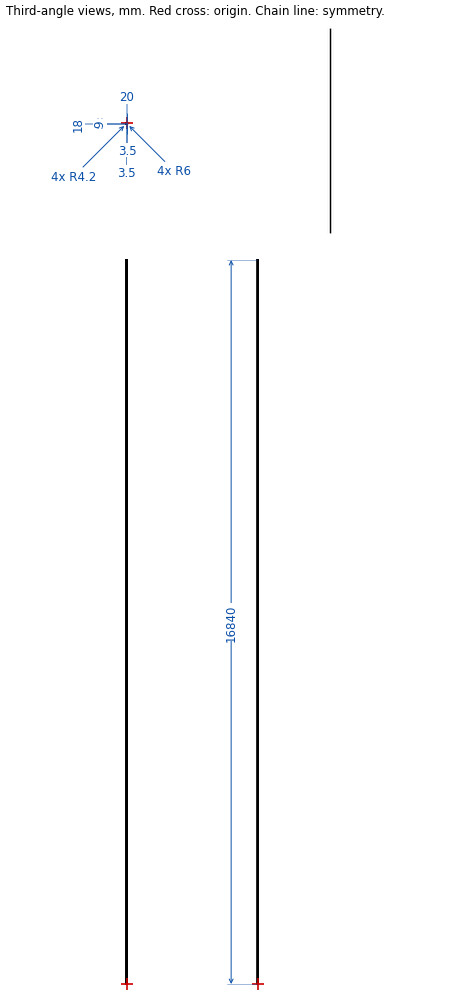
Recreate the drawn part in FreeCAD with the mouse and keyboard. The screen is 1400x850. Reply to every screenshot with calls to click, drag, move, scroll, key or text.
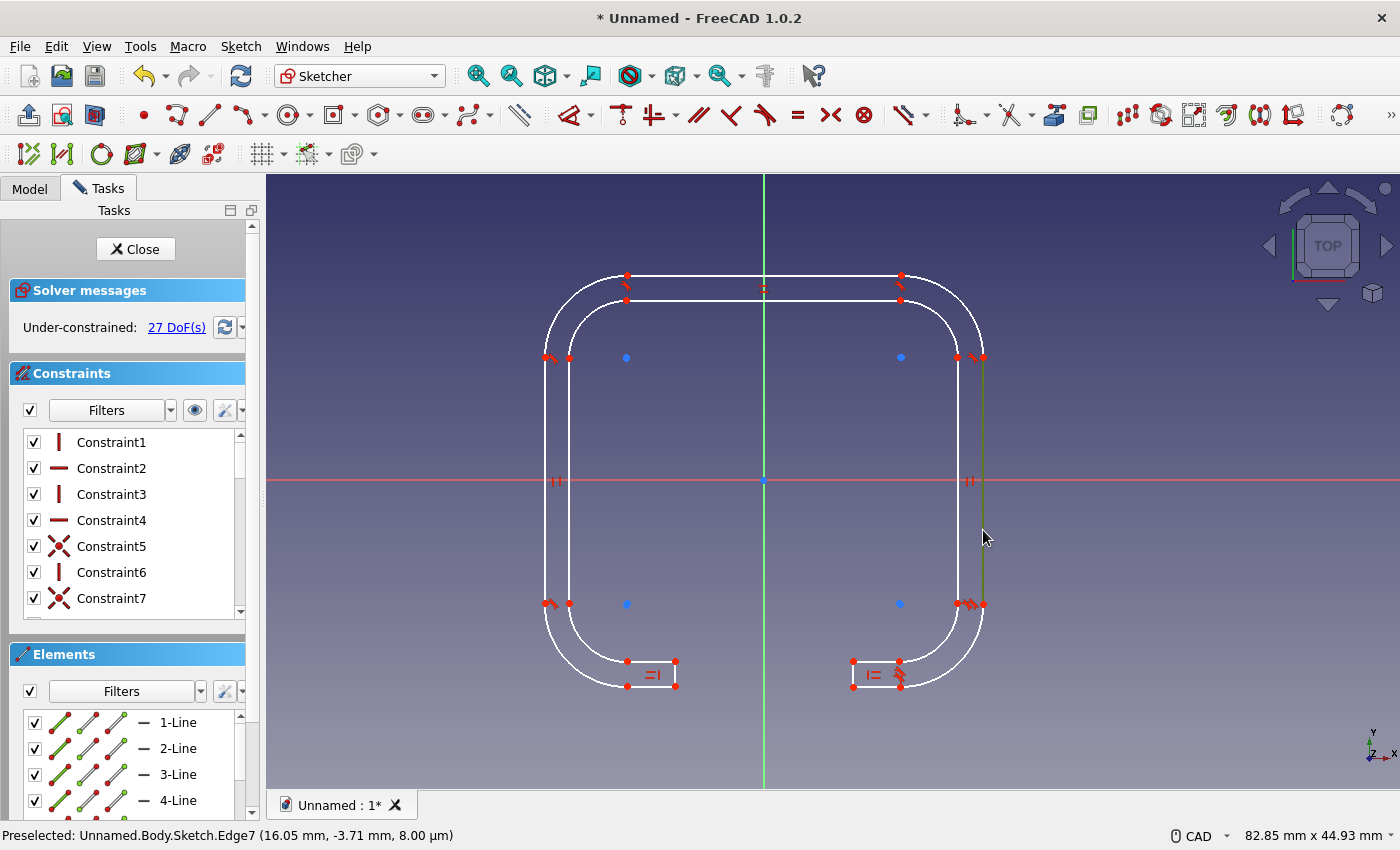
click(974, 321)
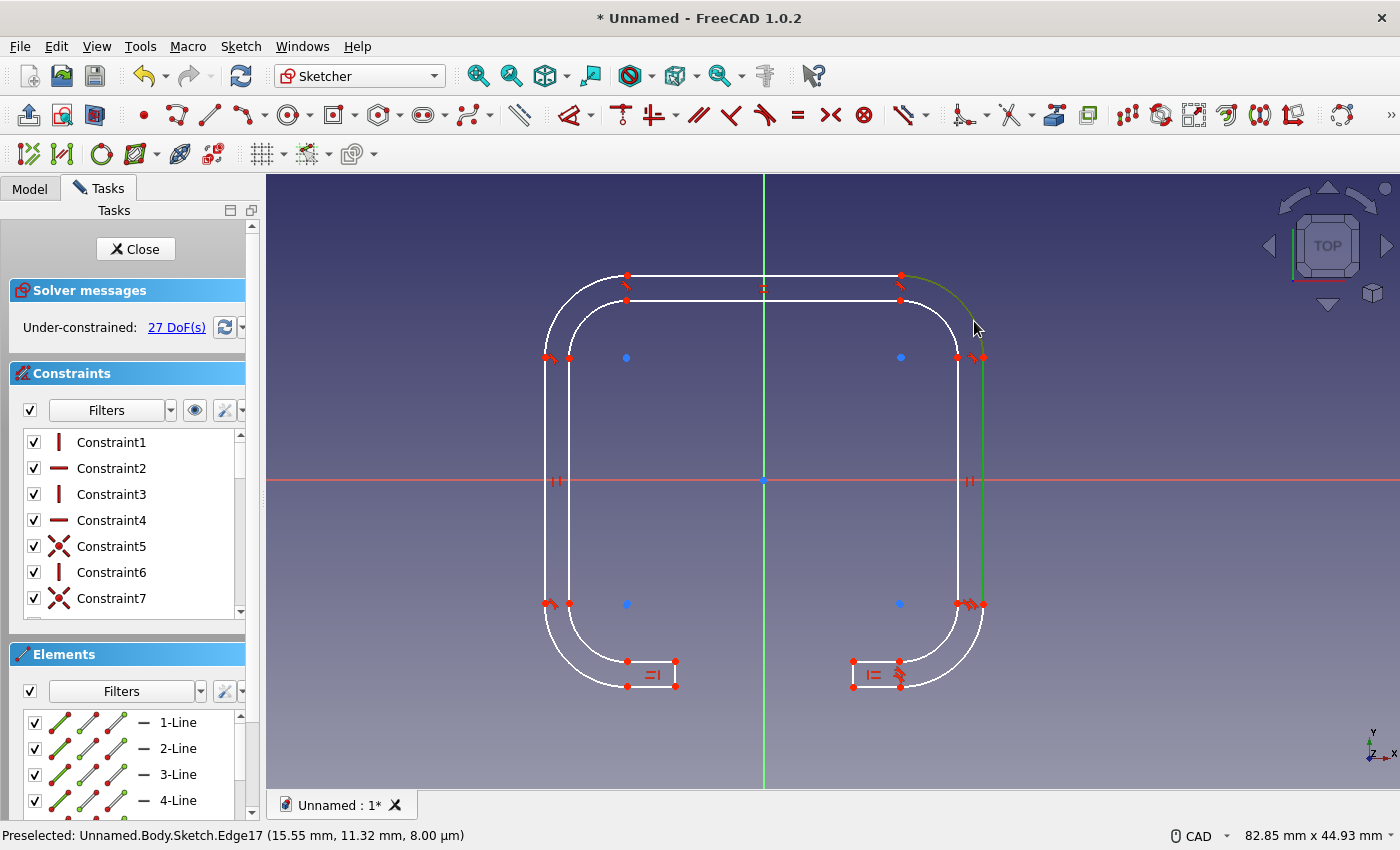
click(765, 116)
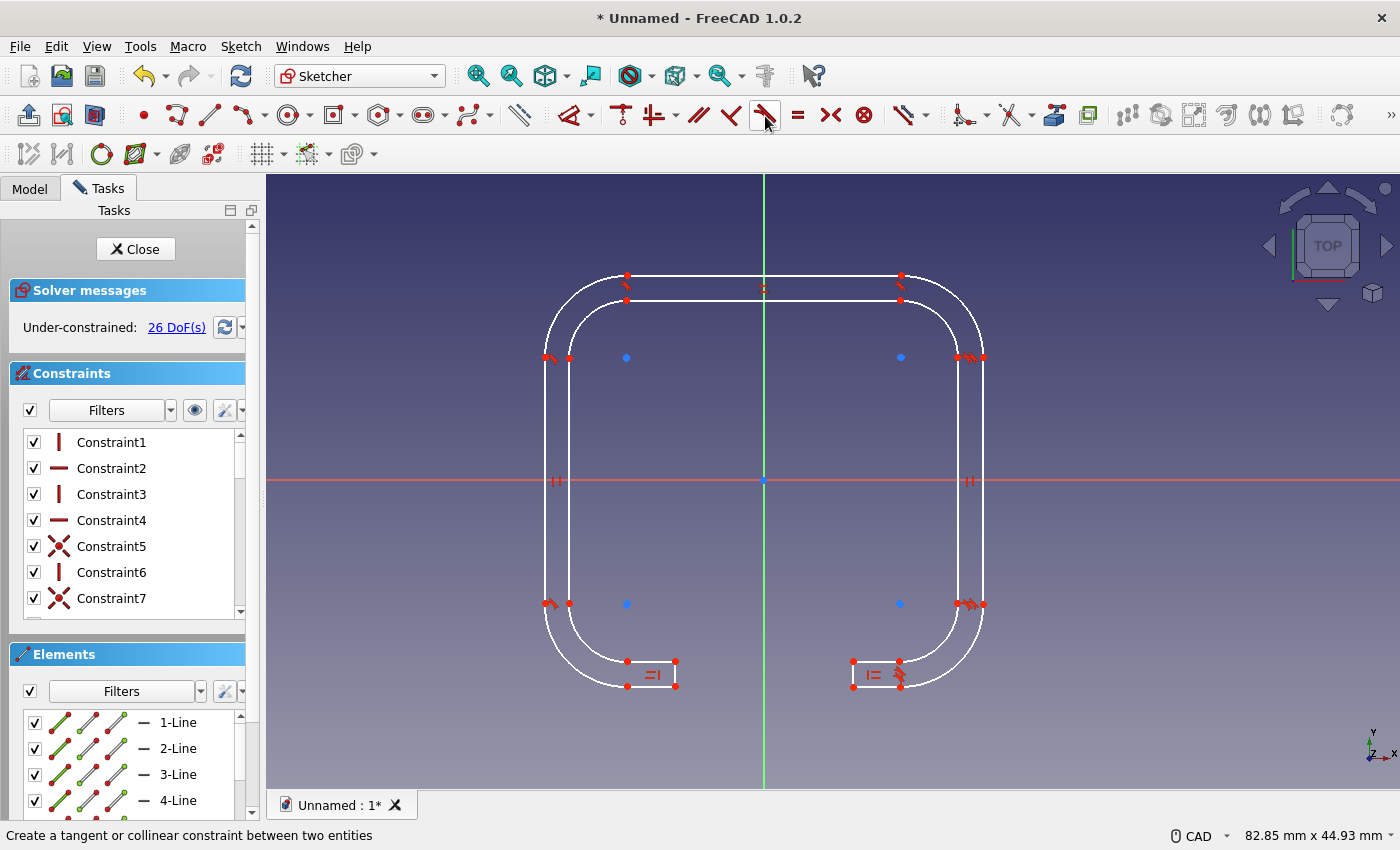
click(819, 276)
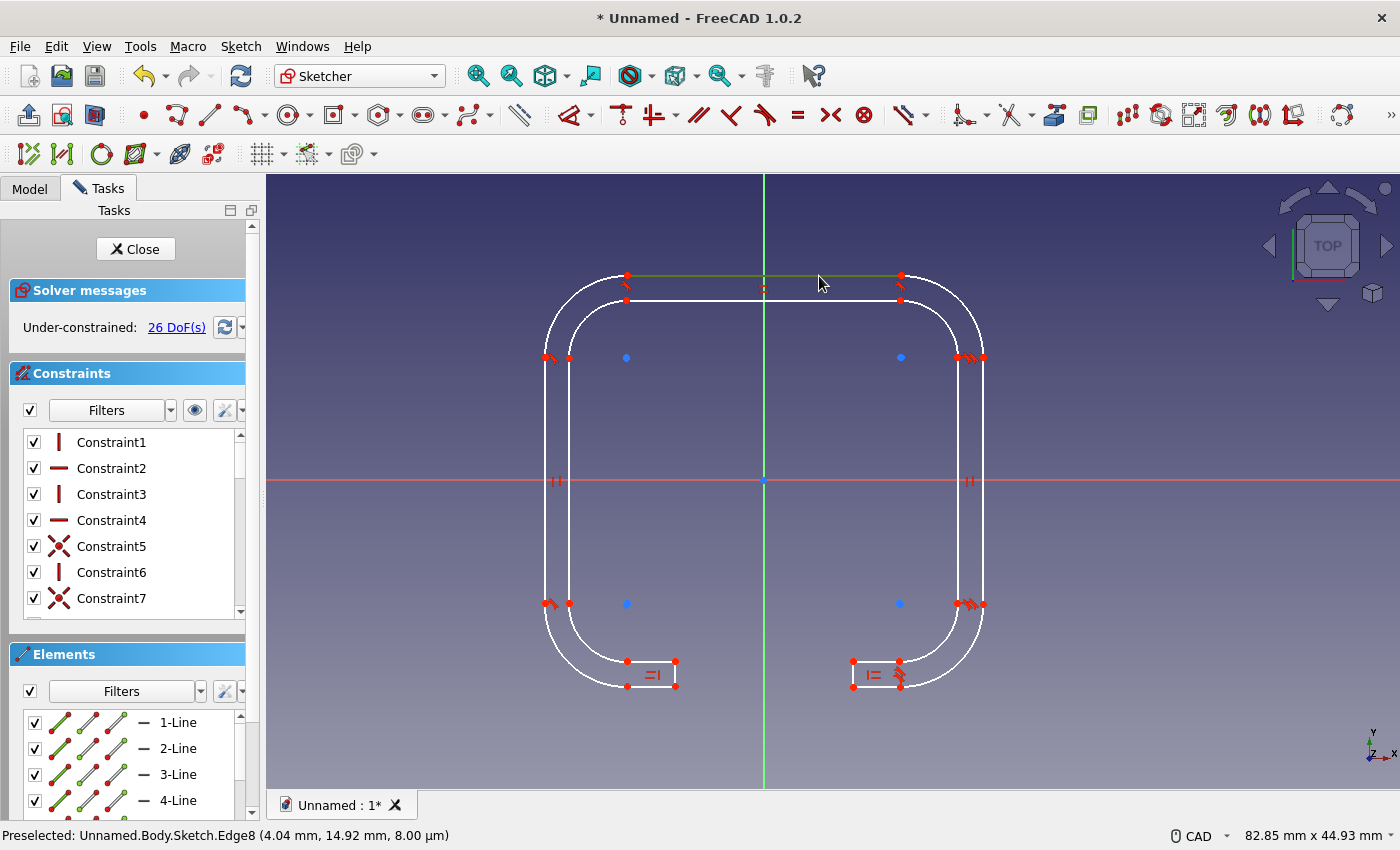
click(974, 321)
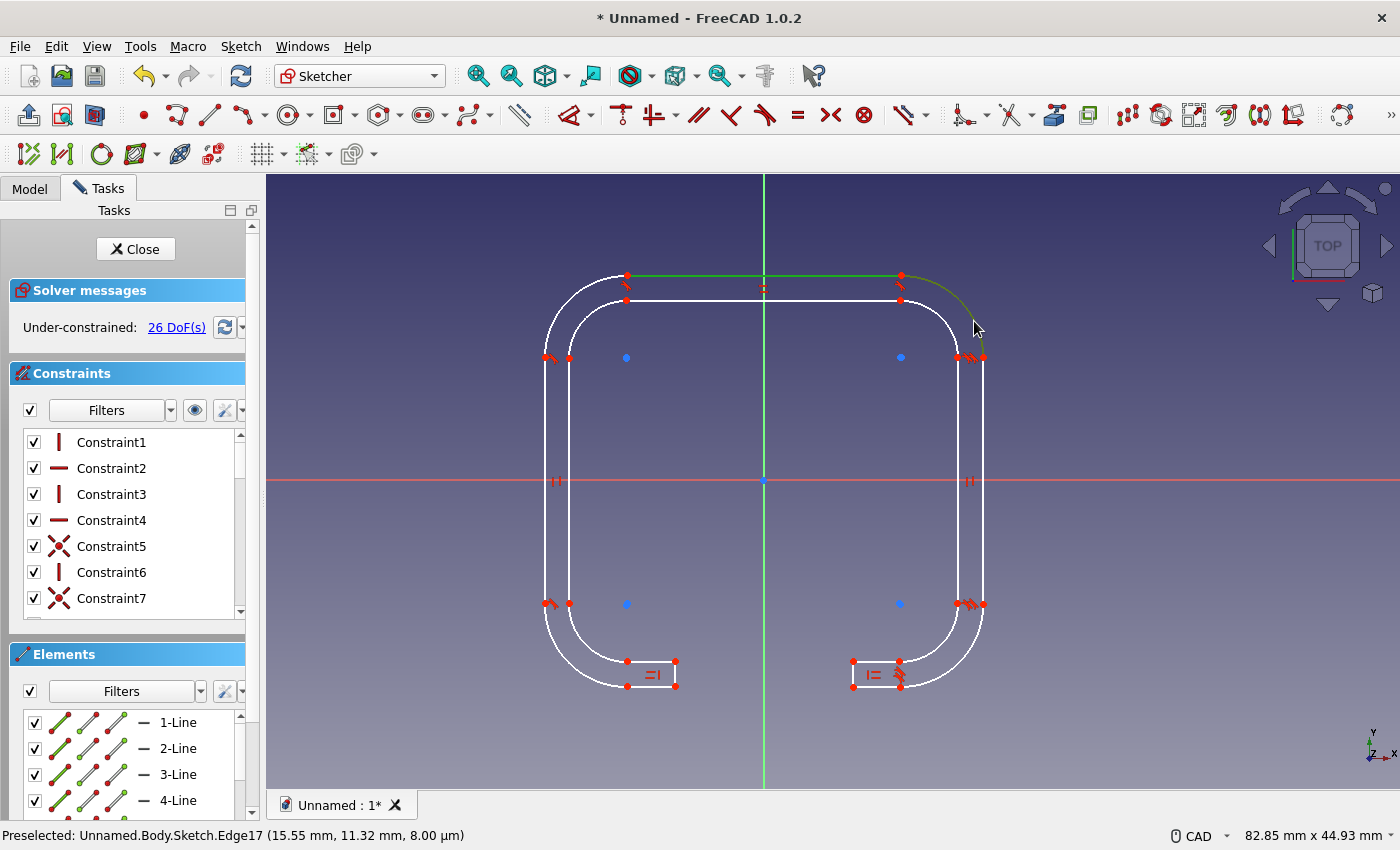
click(765, 116)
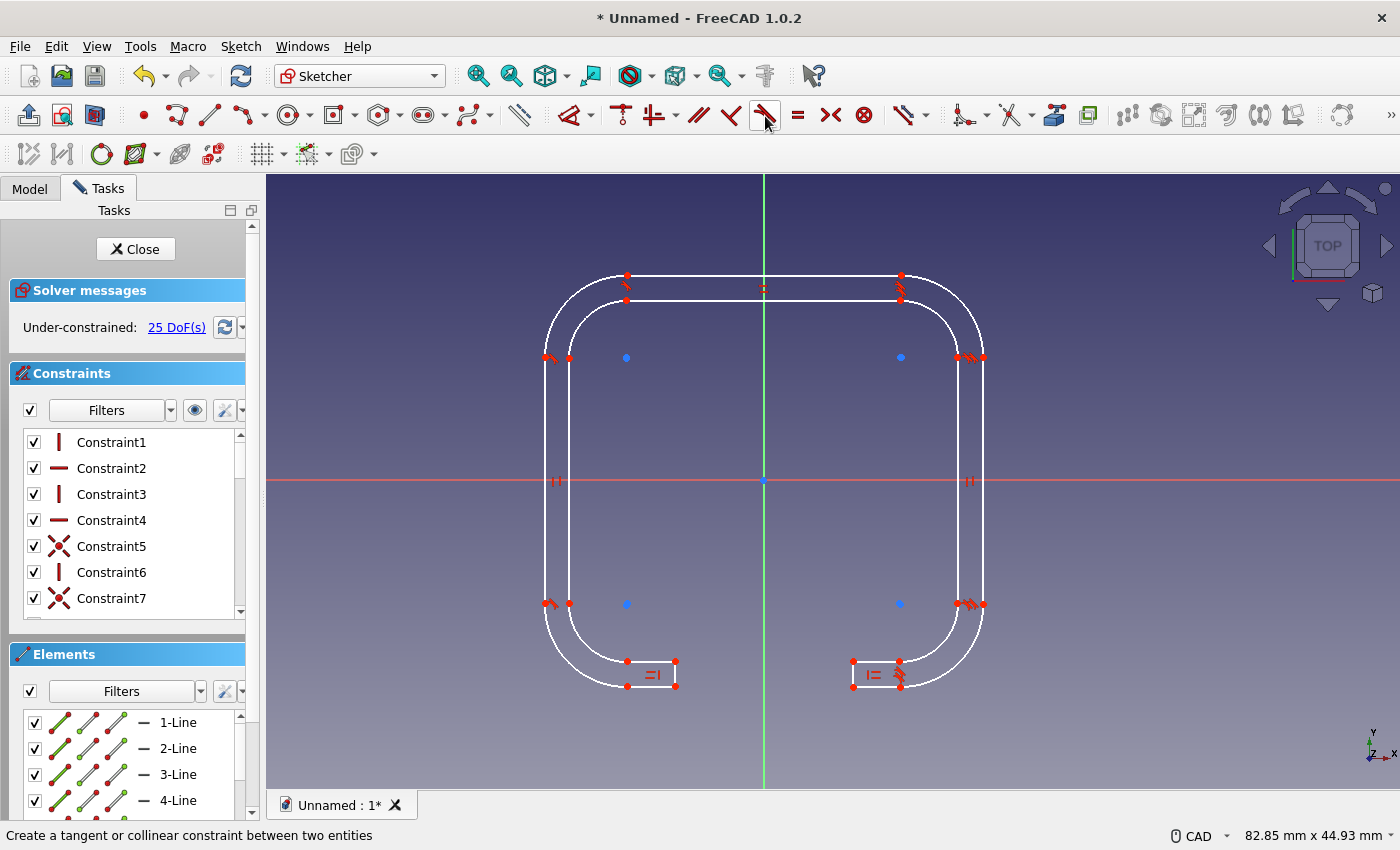
click(819, 276)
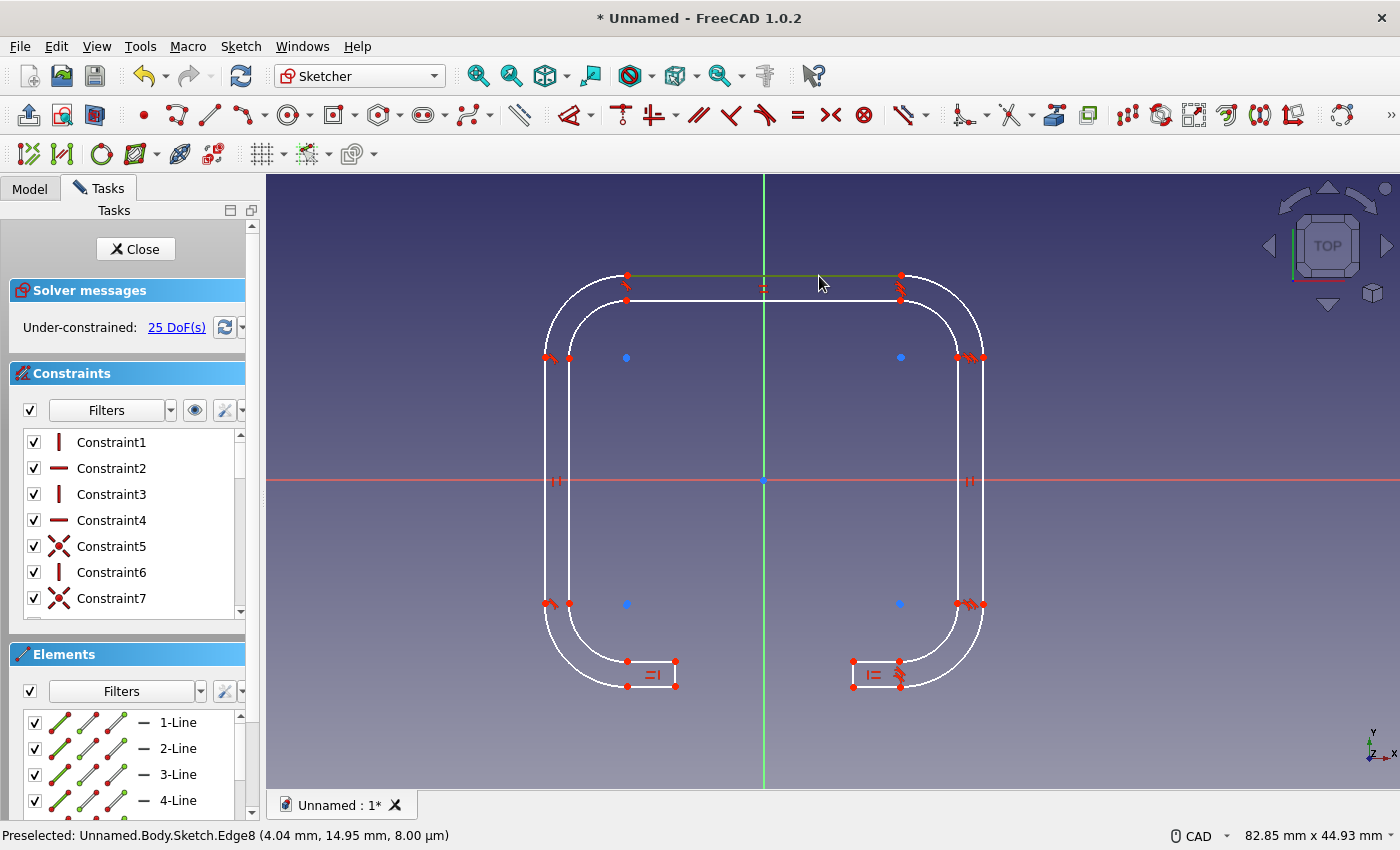
click(590, 285)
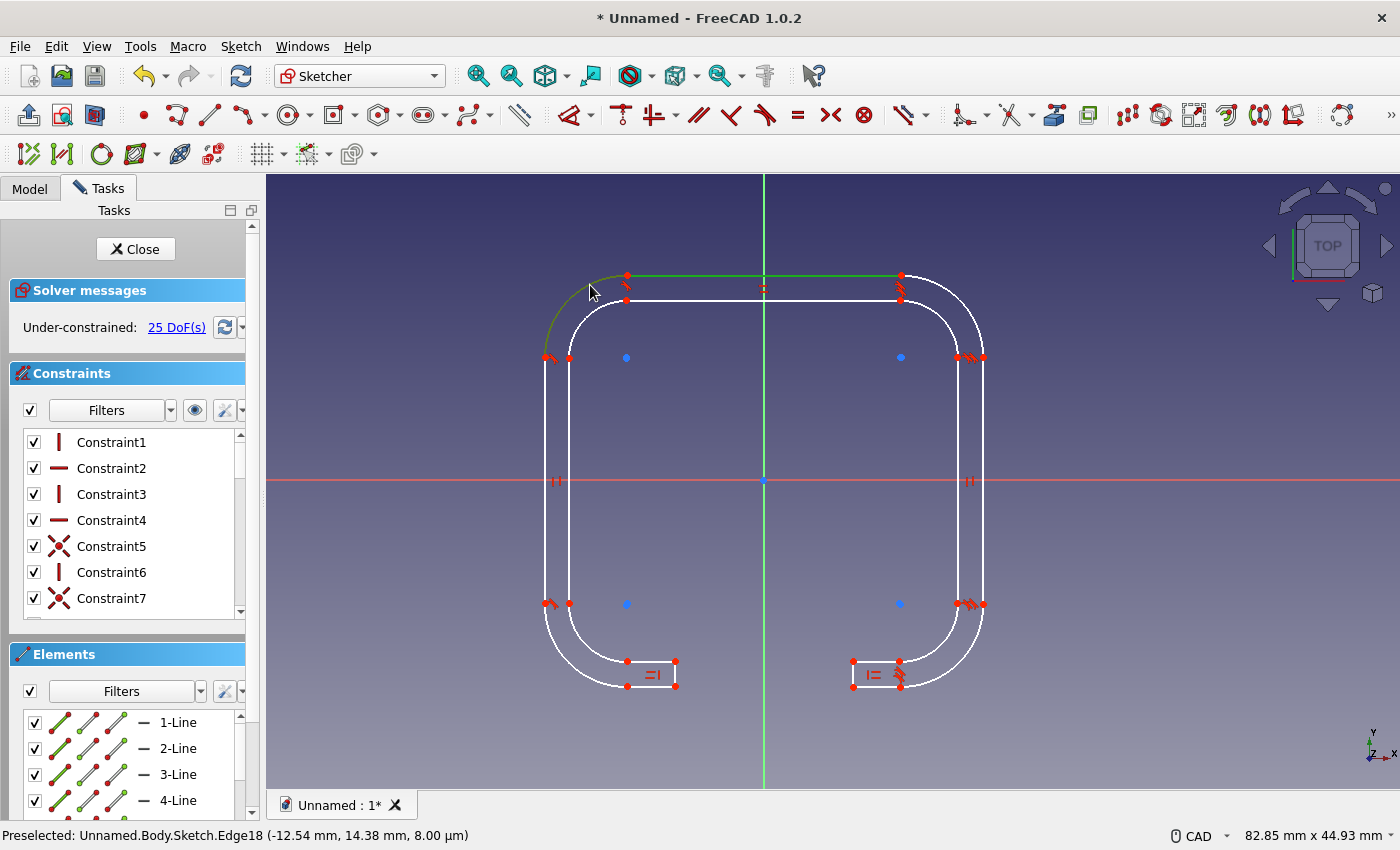
click(765, 116)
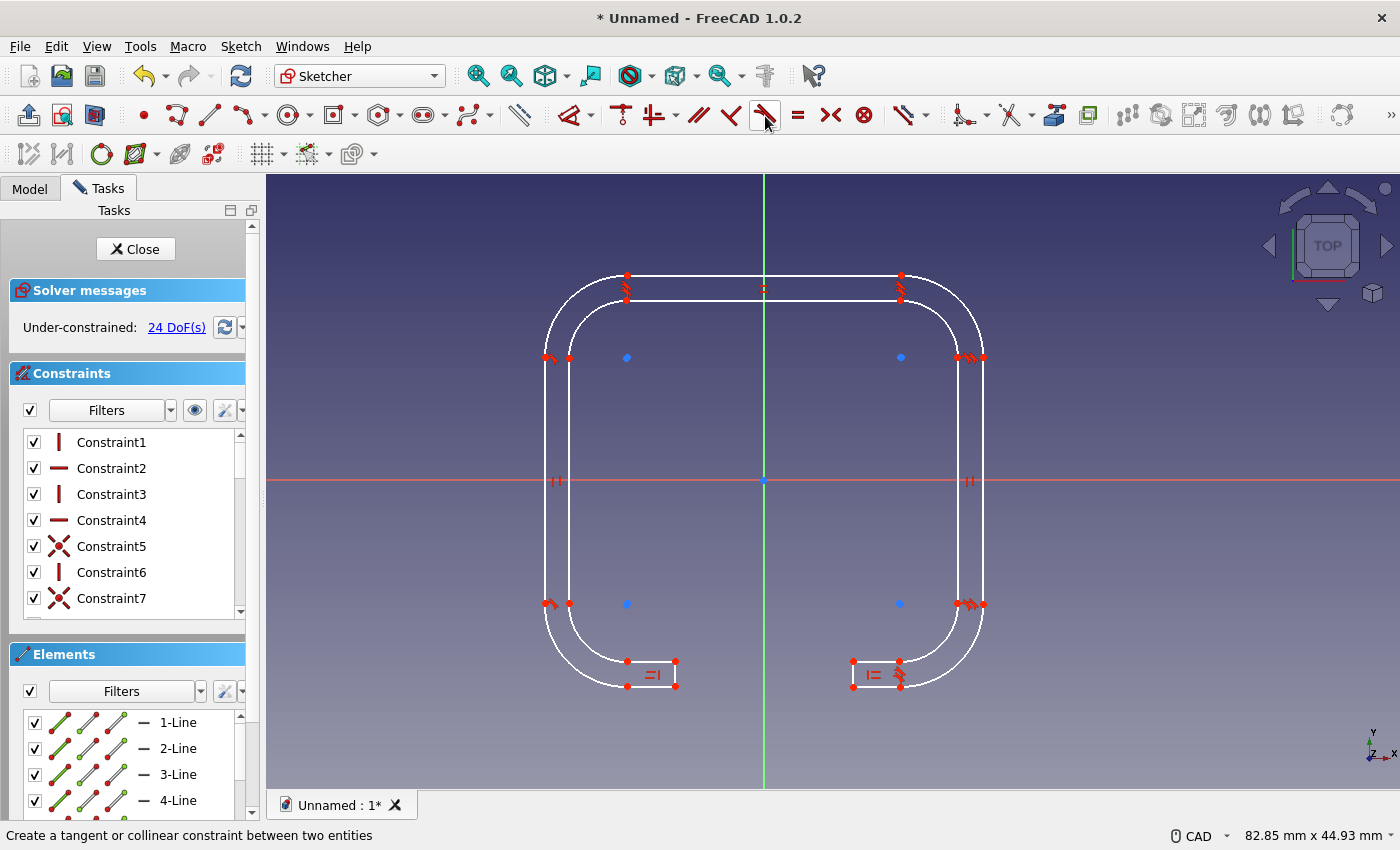
click(545, 432)